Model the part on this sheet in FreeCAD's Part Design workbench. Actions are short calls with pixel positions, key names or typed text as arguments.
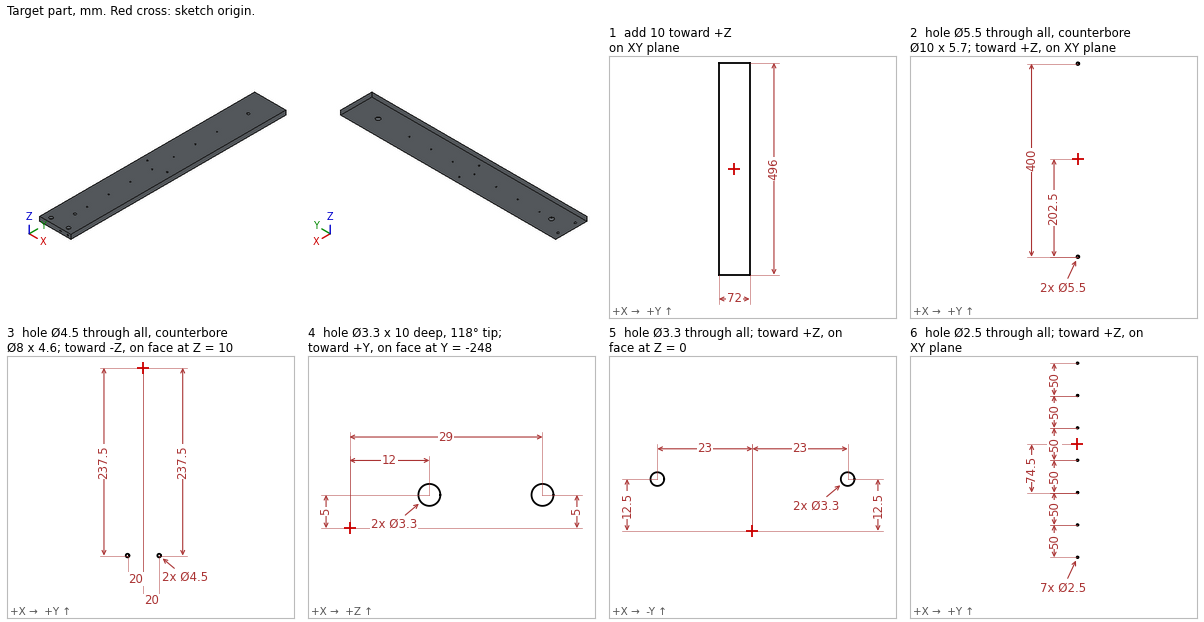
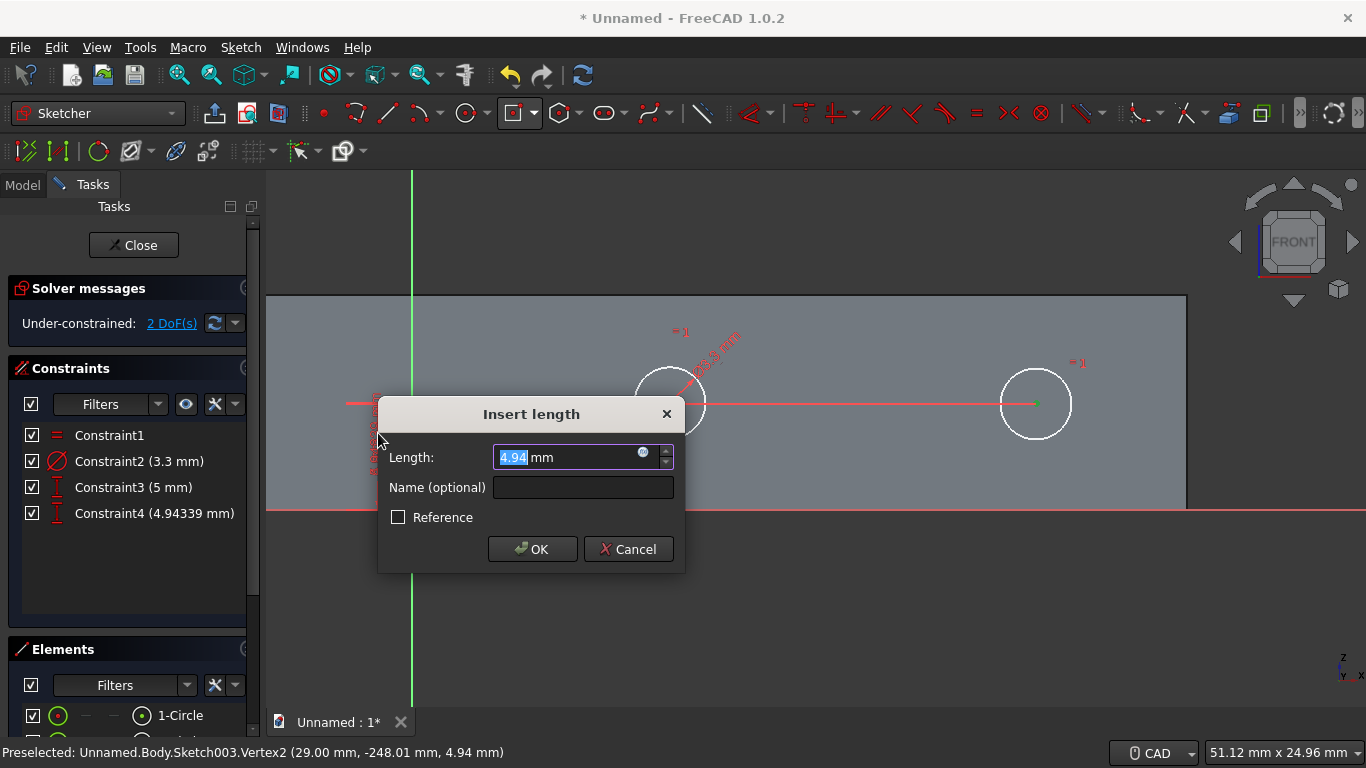
text(5)
key(Return)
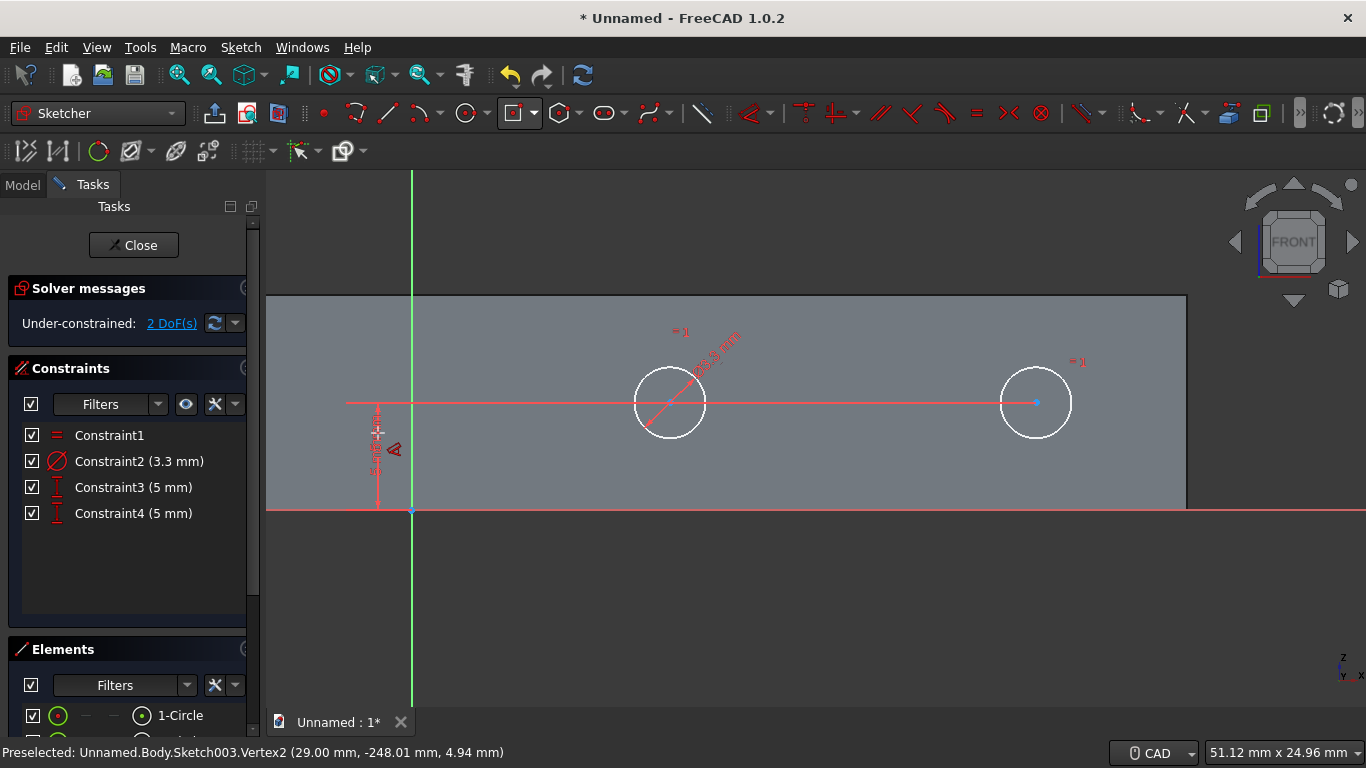
click(670, 403)
click(541, 544)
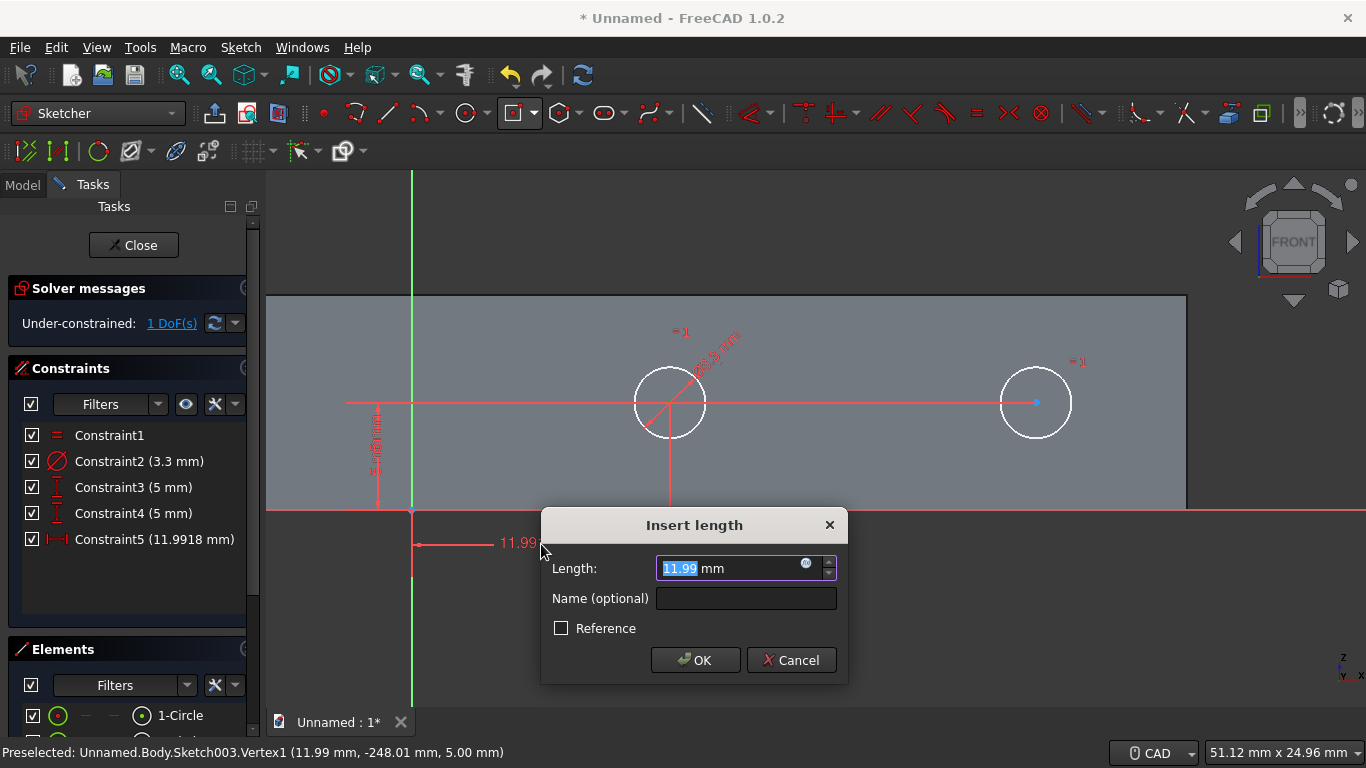
text(12)
key(Return)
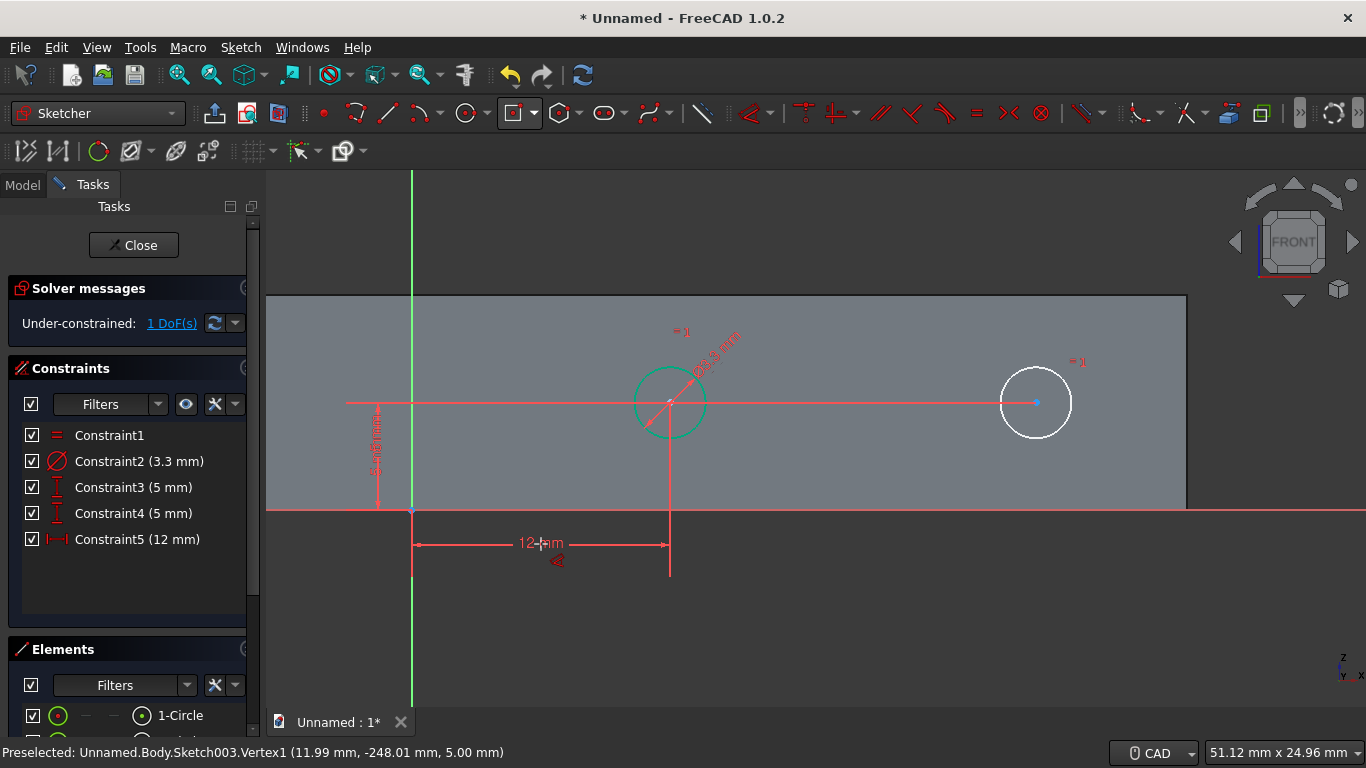
click(1036, 403)
click(724, 544)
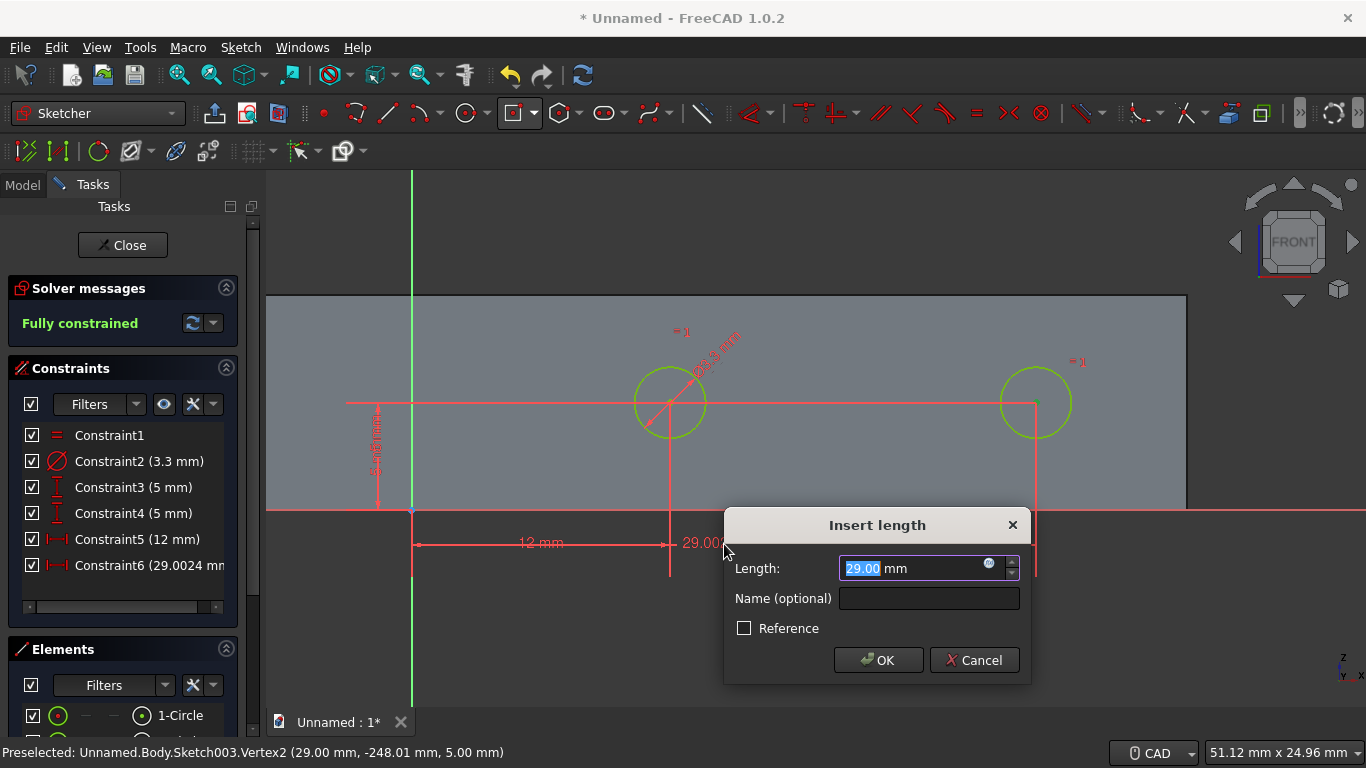
text(29)
key(Return)
key(Escape)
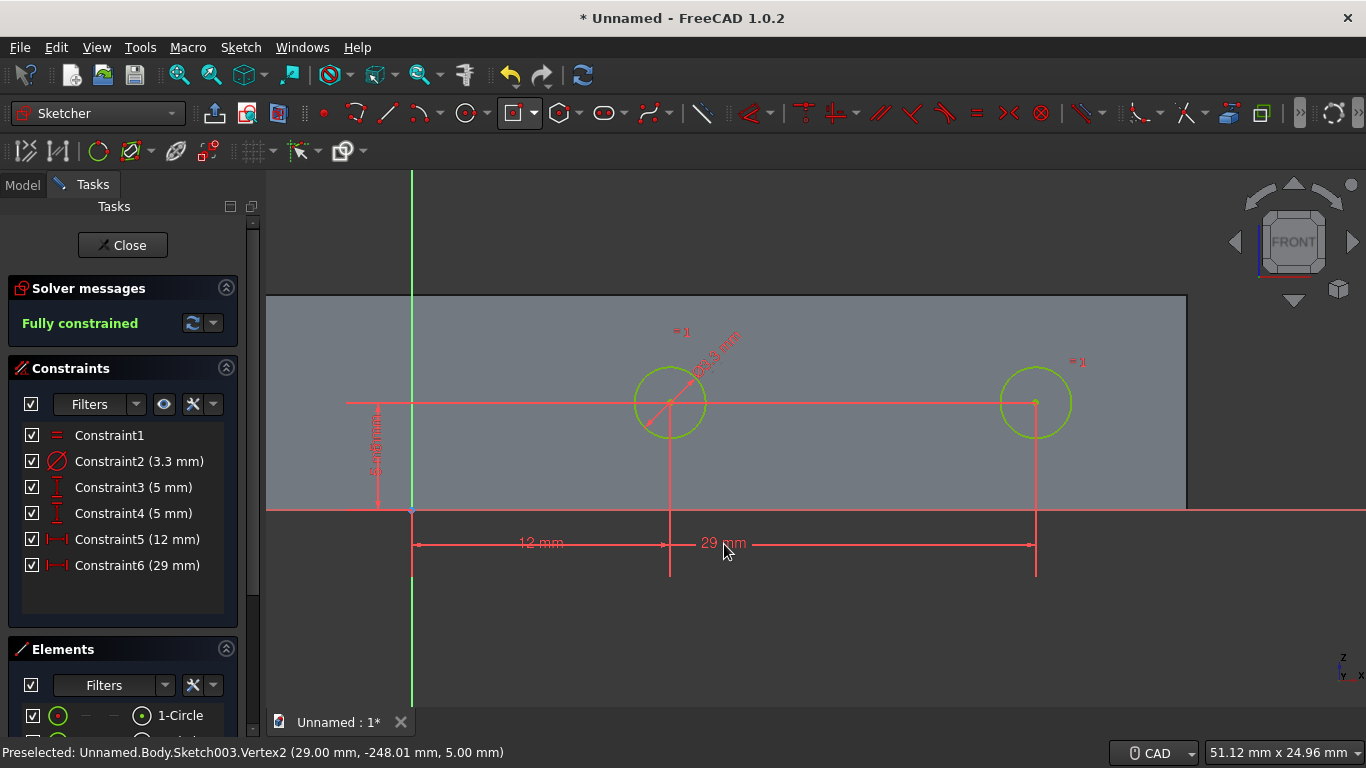
click(123, 245)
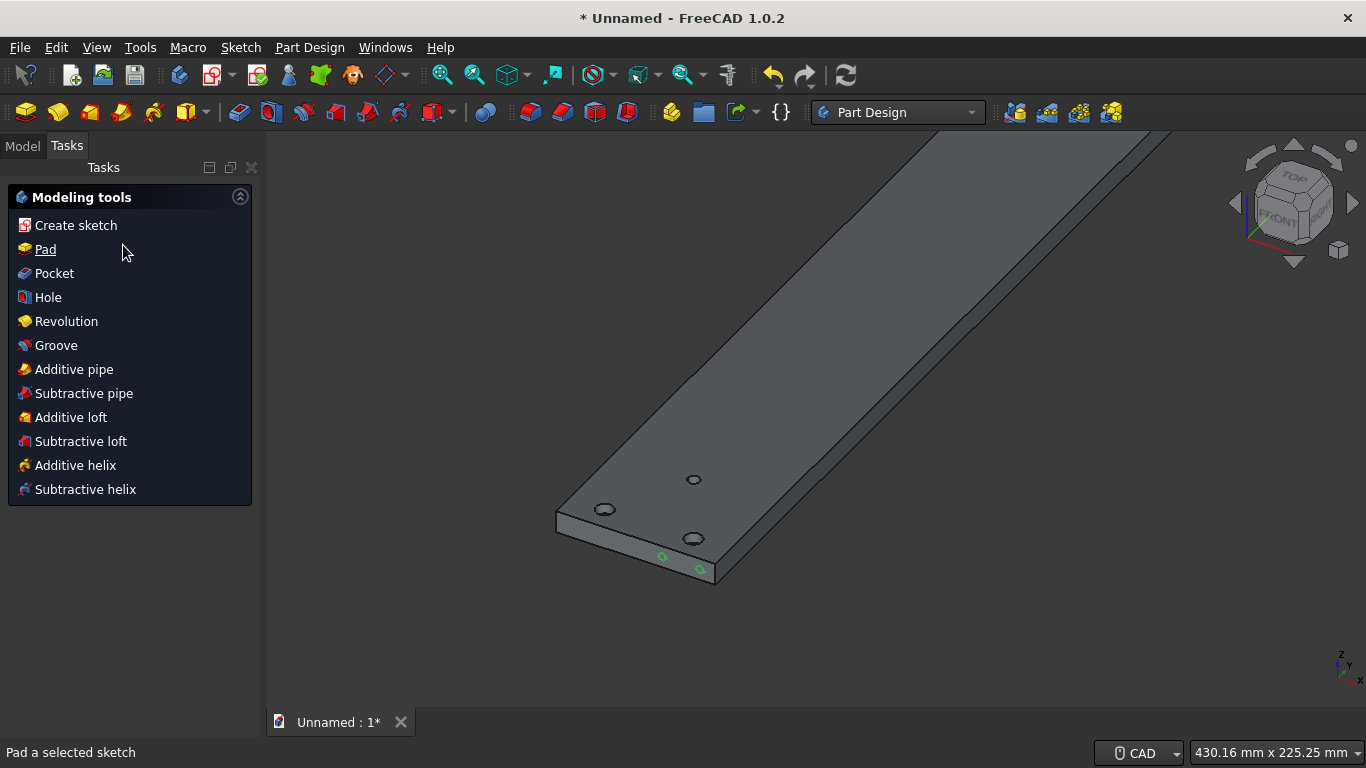
click(272, 112)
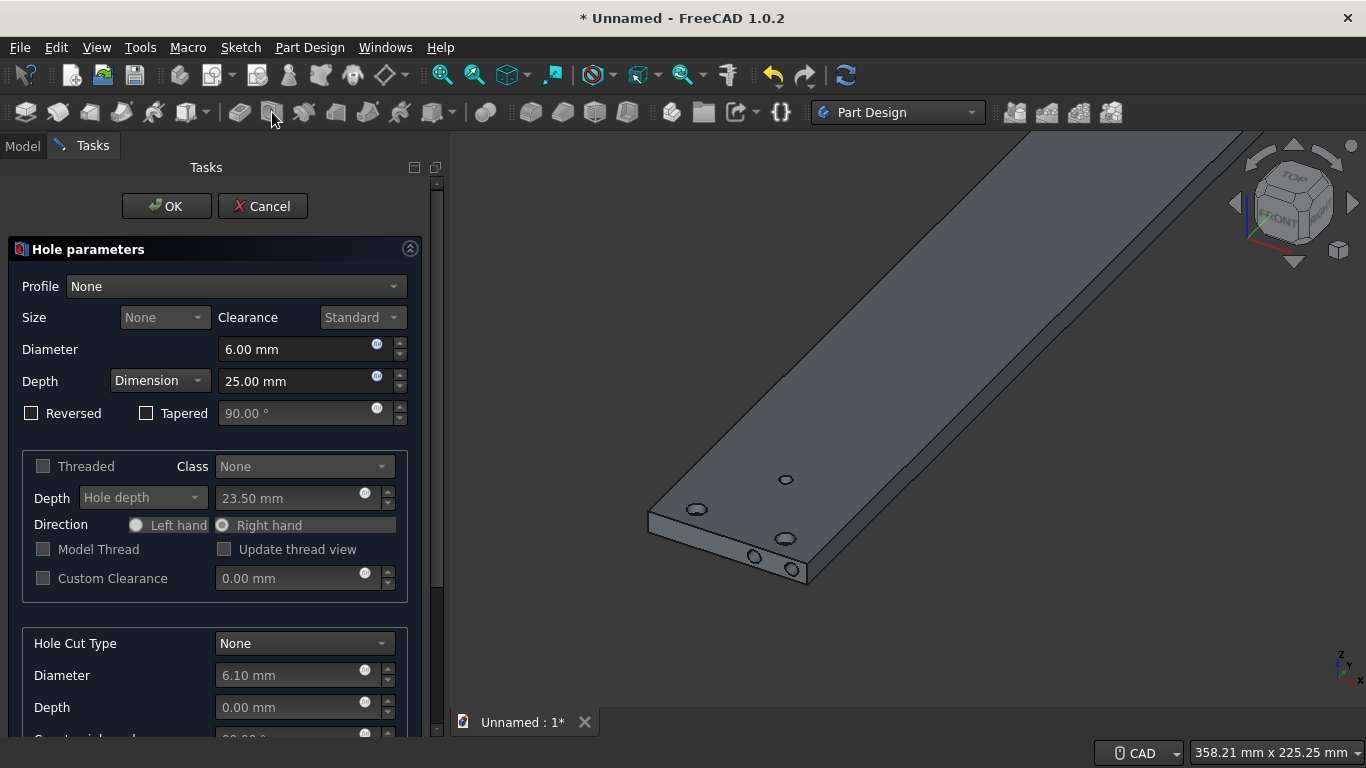
triple_click(305, 349)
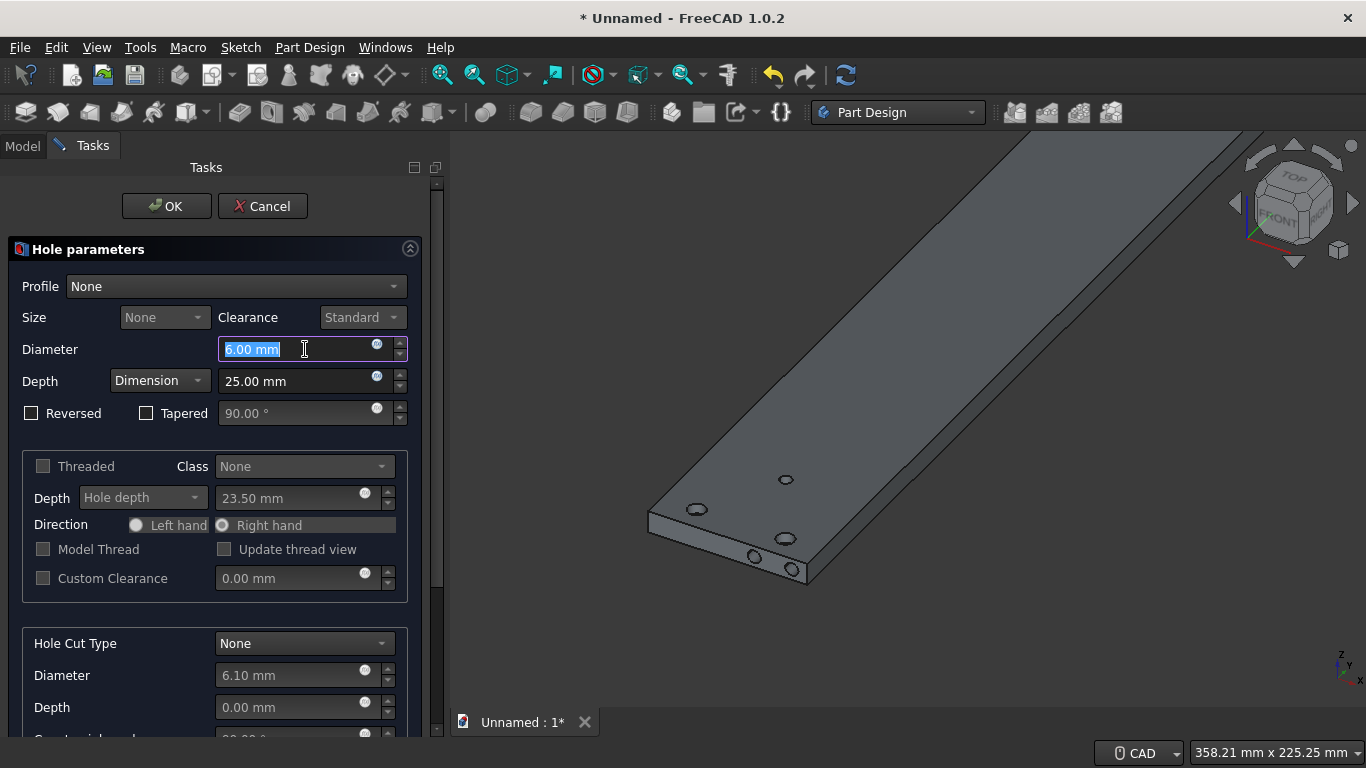
text(3.3)
key(Tab)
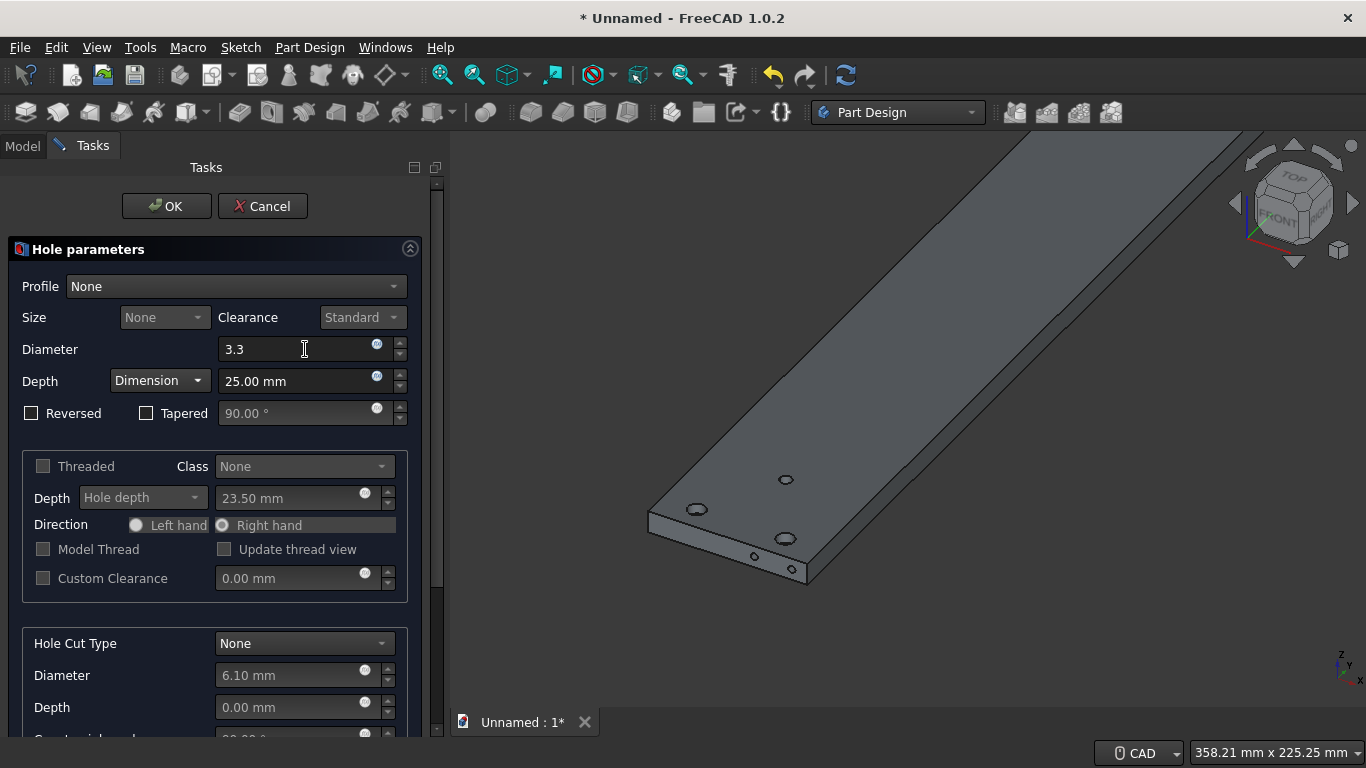
triple_click(305, 381)